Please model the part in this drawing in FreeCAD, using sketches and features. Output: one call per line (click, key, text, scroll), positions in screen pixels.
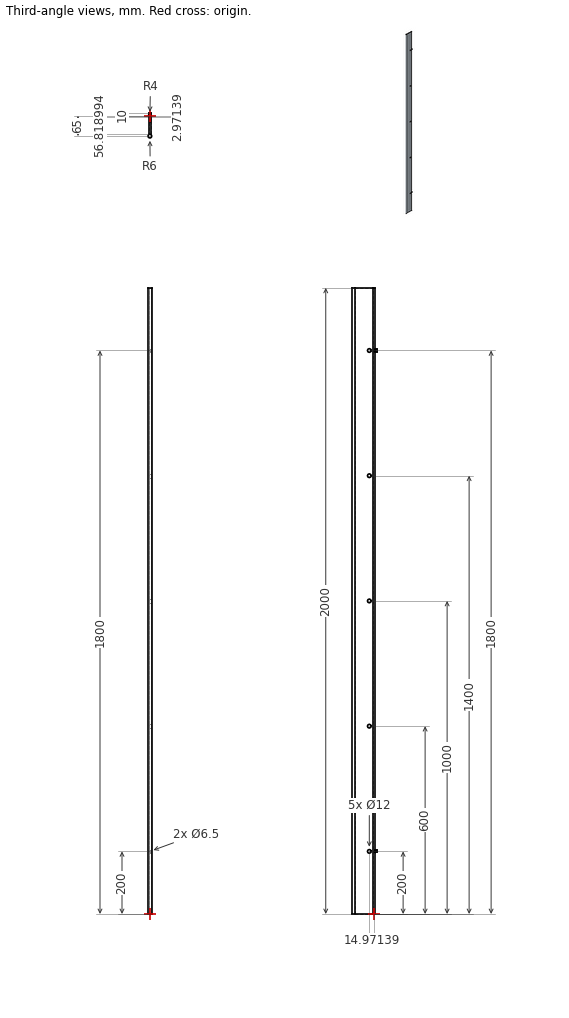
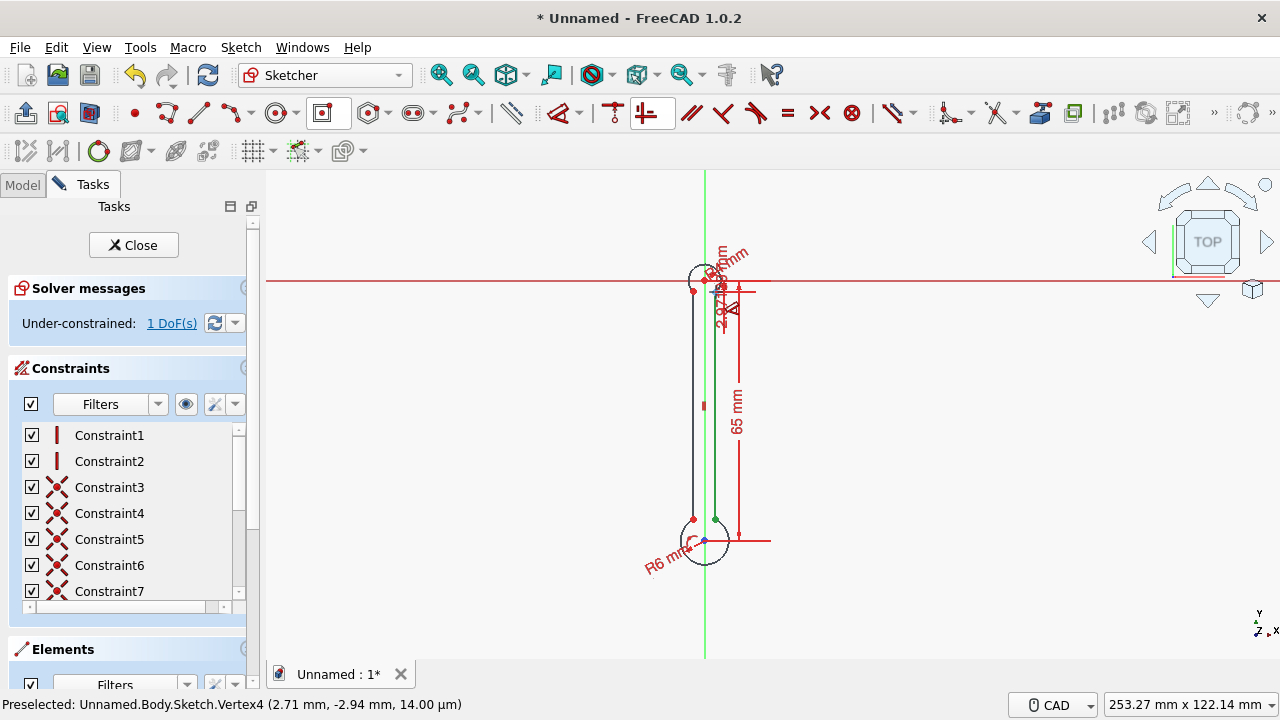
scroll(693, 360, up, 2)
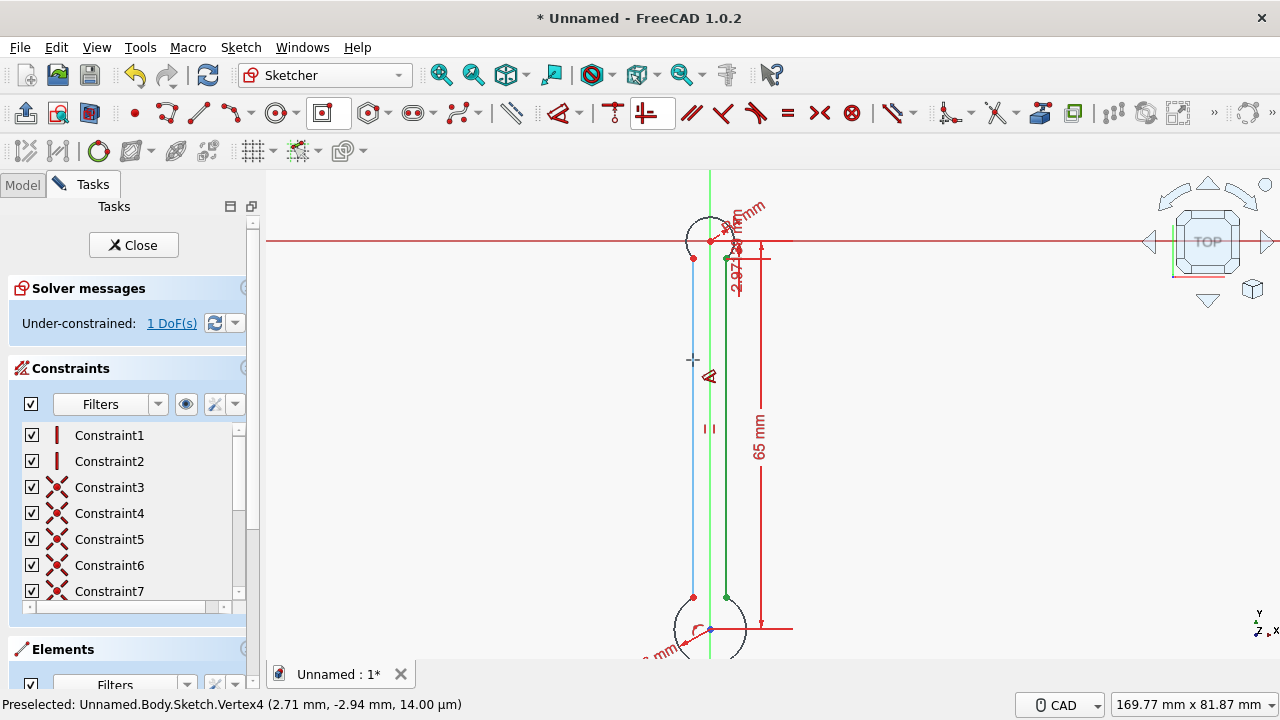
click(693, 360)
click(659, 428)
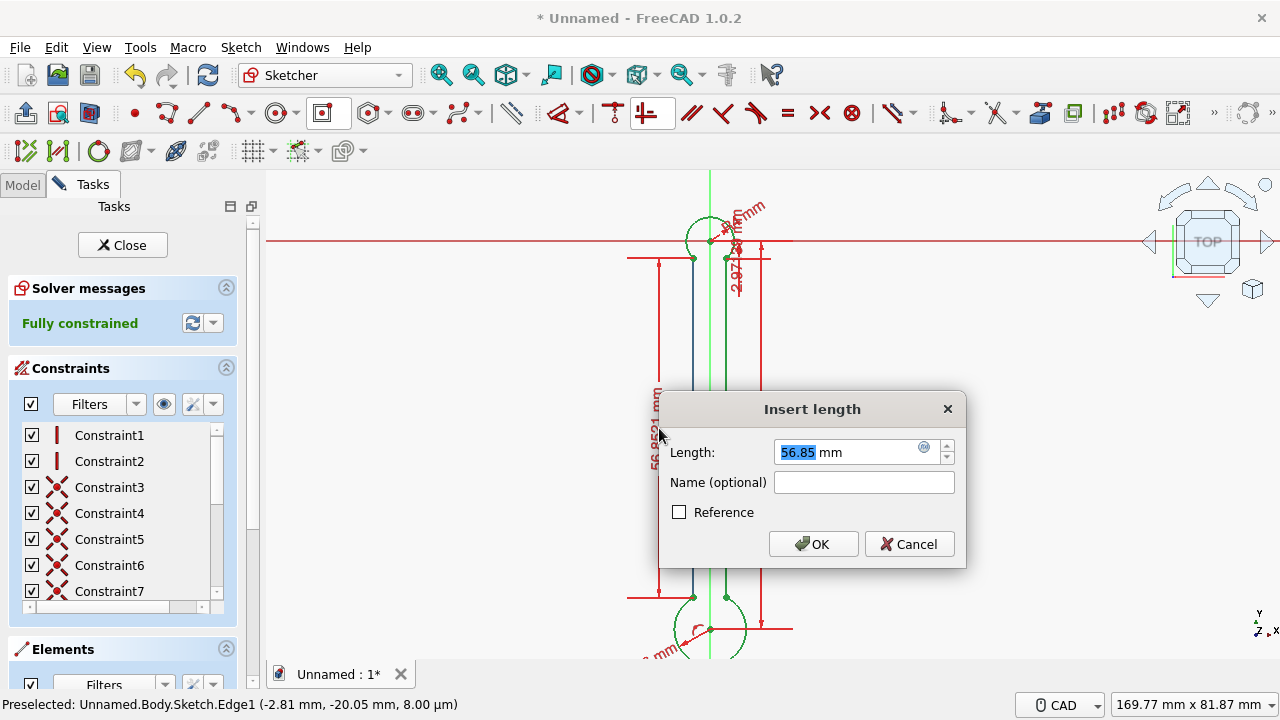
text(56.818994)
key(Return)
key(Escape)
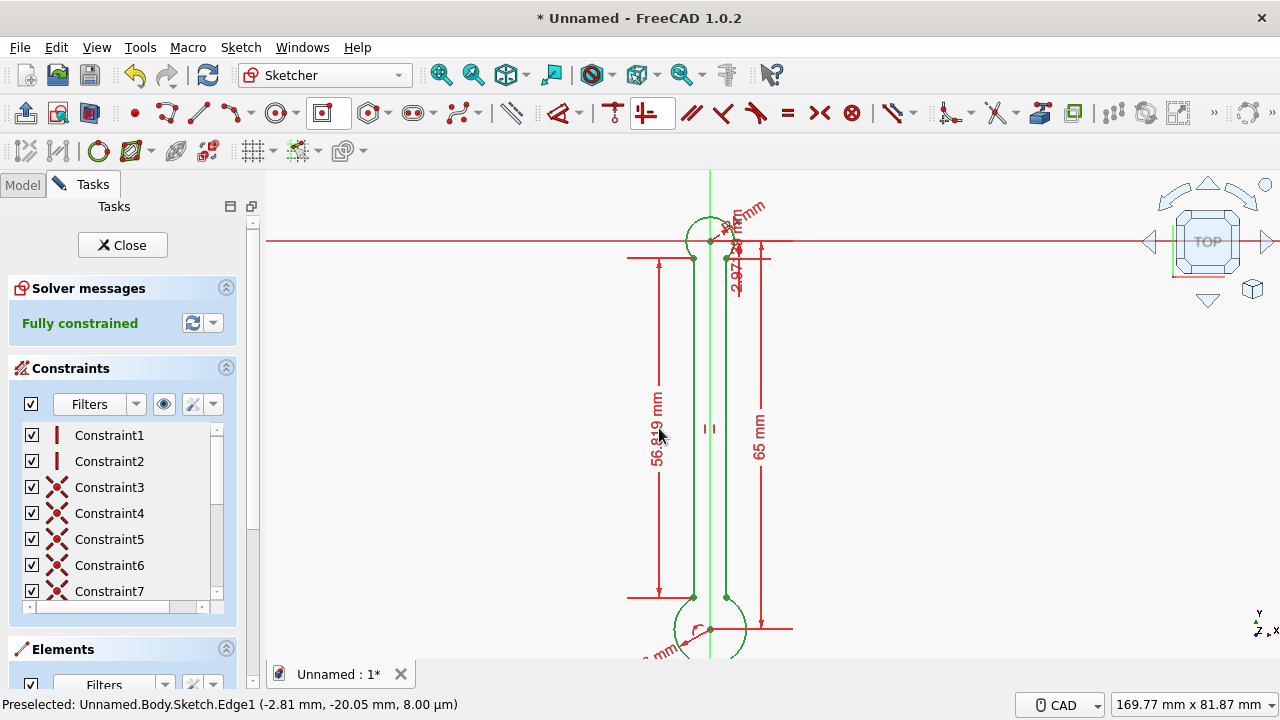
click(123, 245)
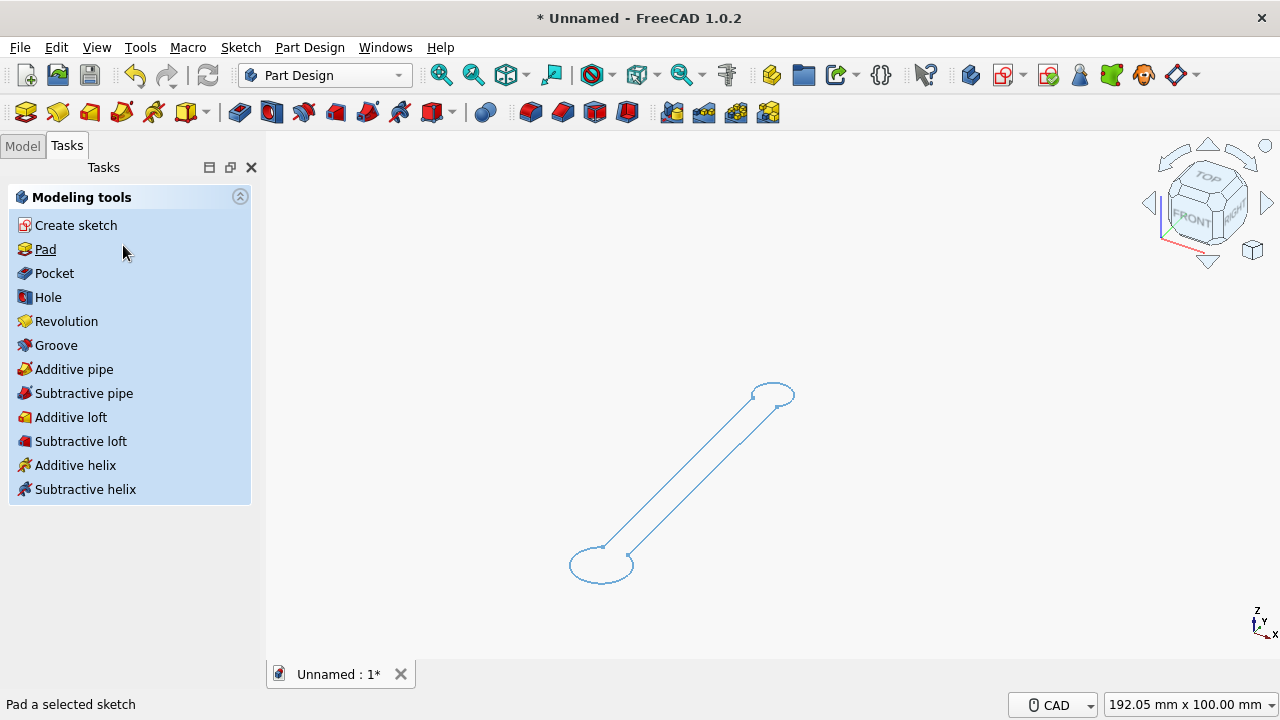
click(26, 112)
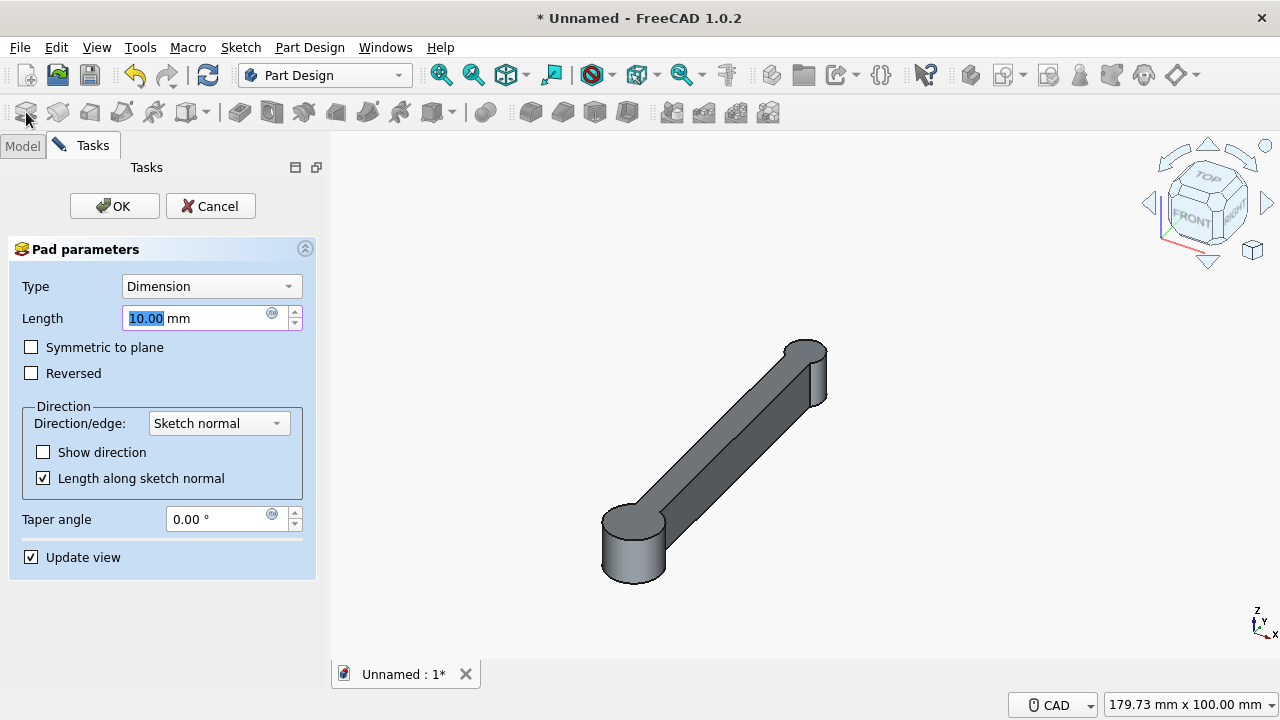
text(2000)
key(Tab)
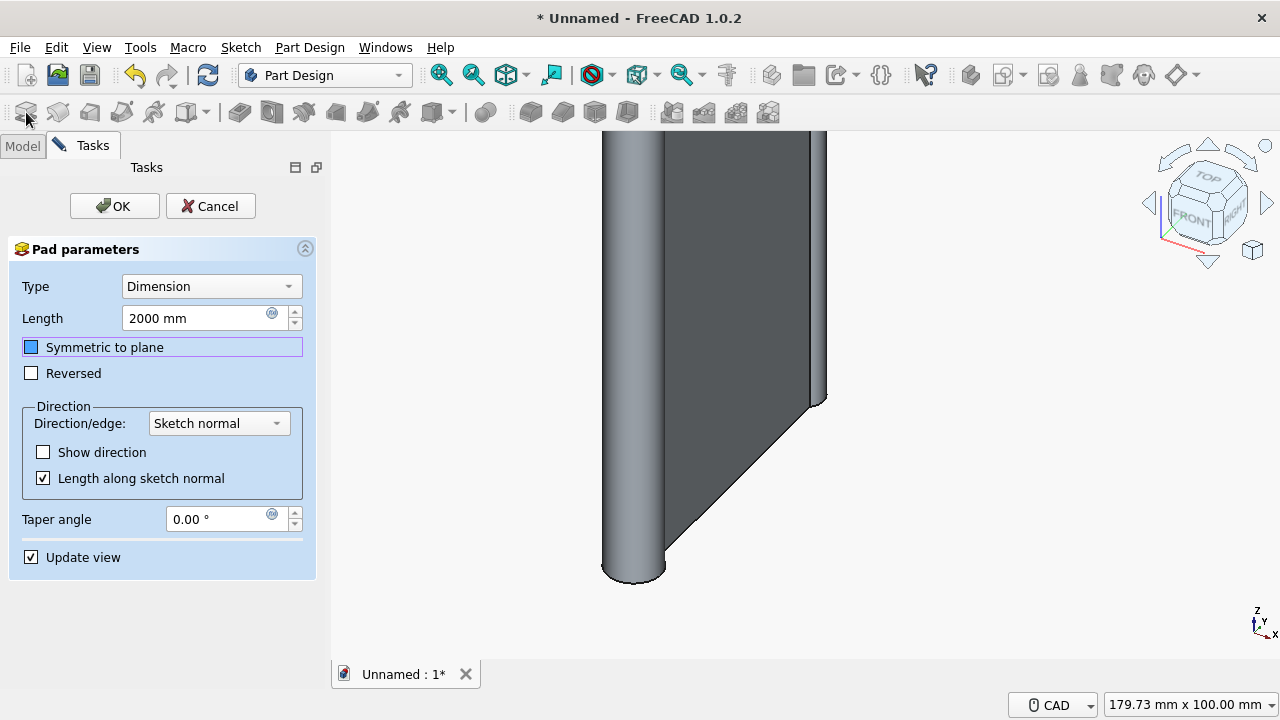
click(115, 206)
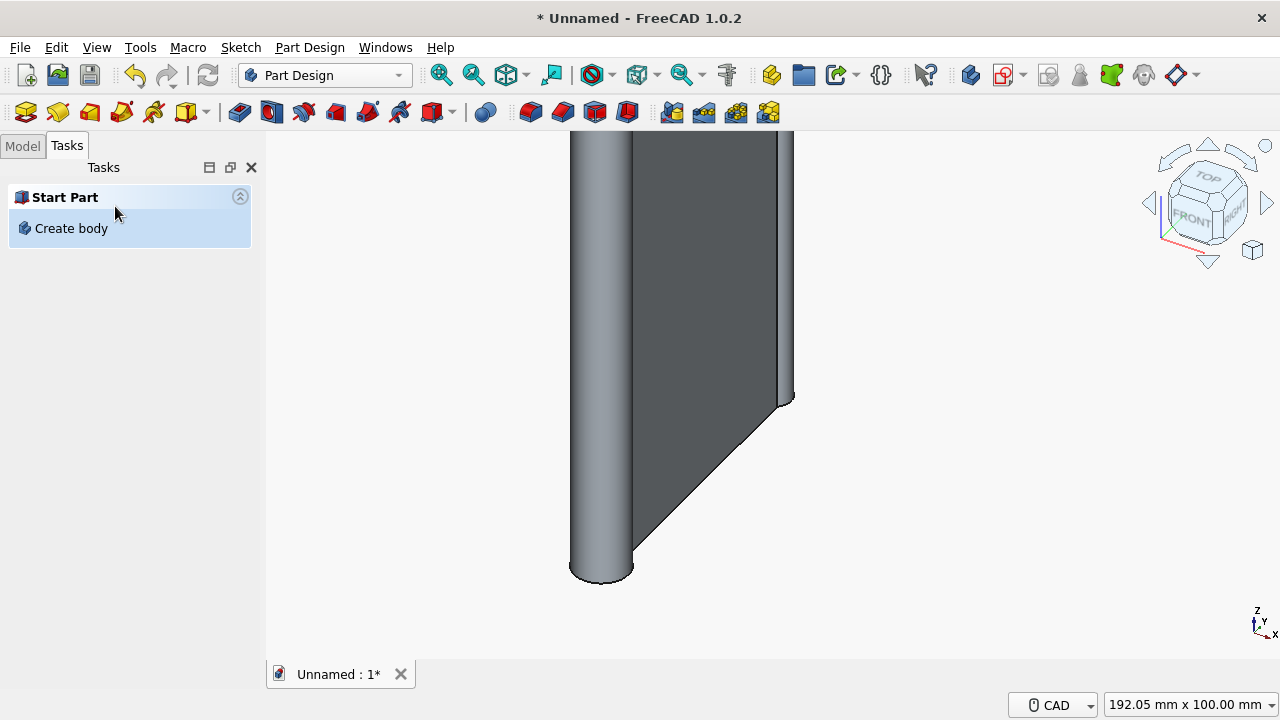
key(v)
key(f)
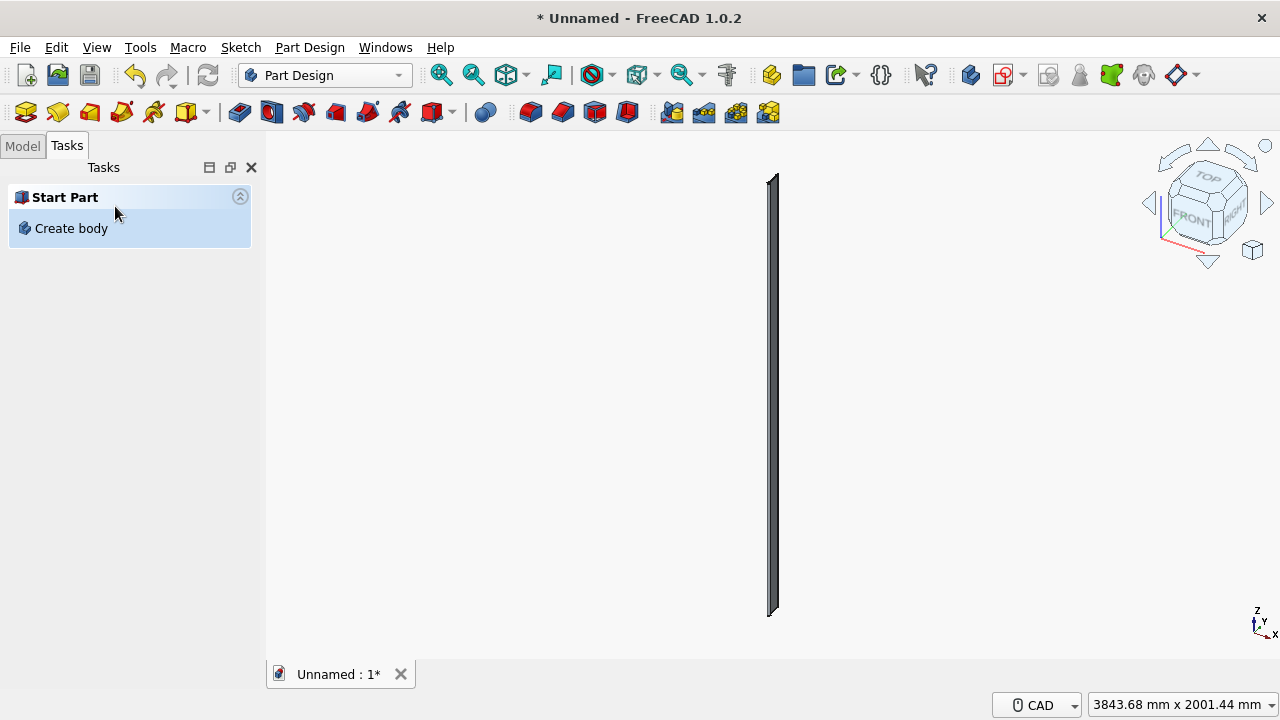
key(0)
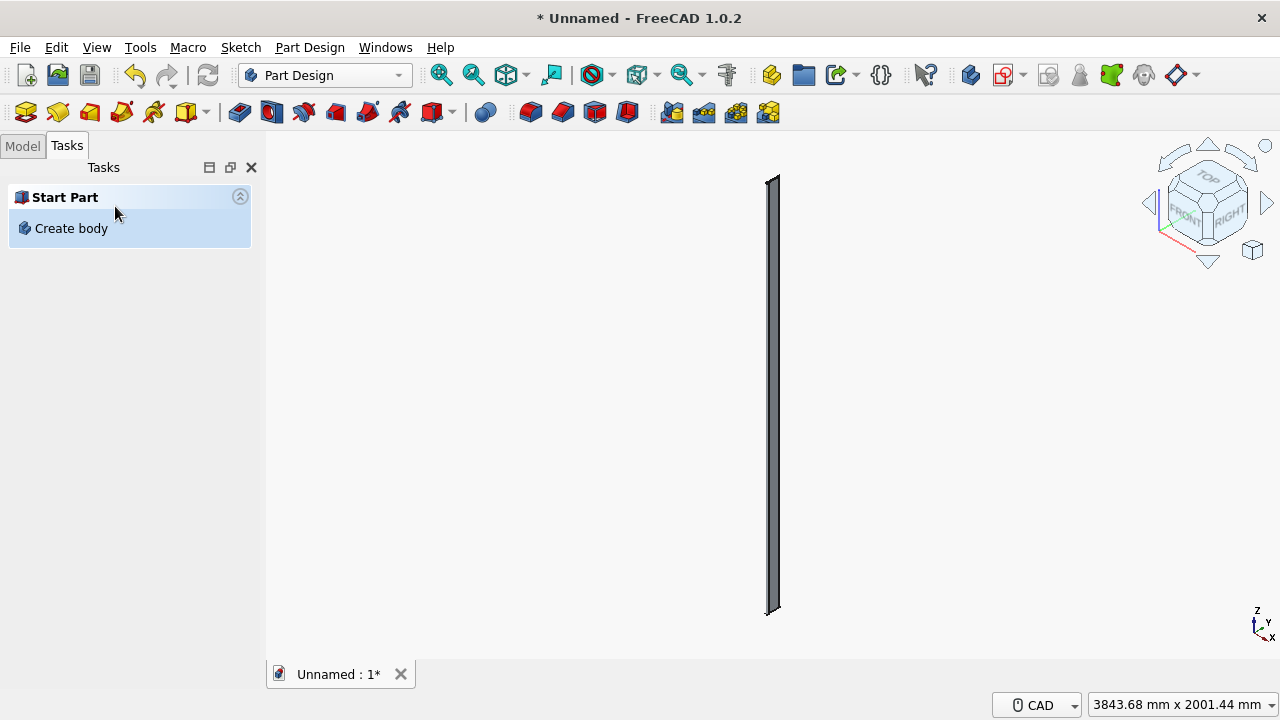
key(3)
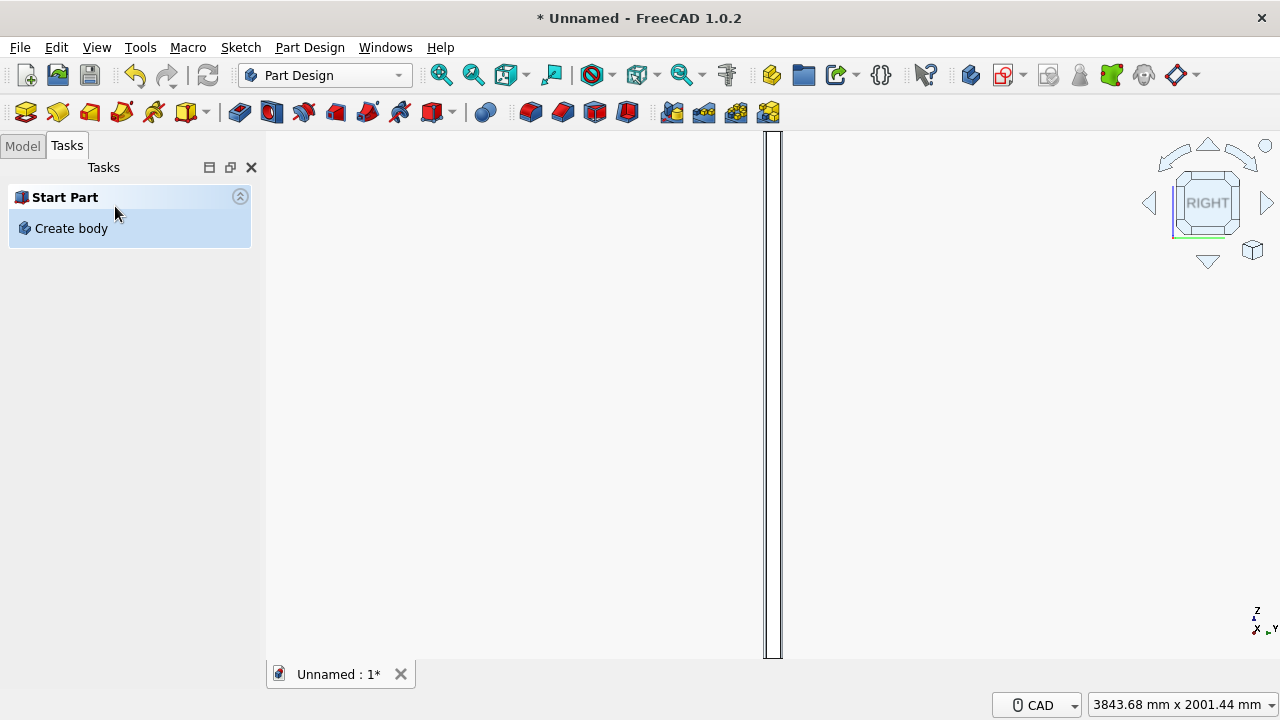
key(v)
key(f)